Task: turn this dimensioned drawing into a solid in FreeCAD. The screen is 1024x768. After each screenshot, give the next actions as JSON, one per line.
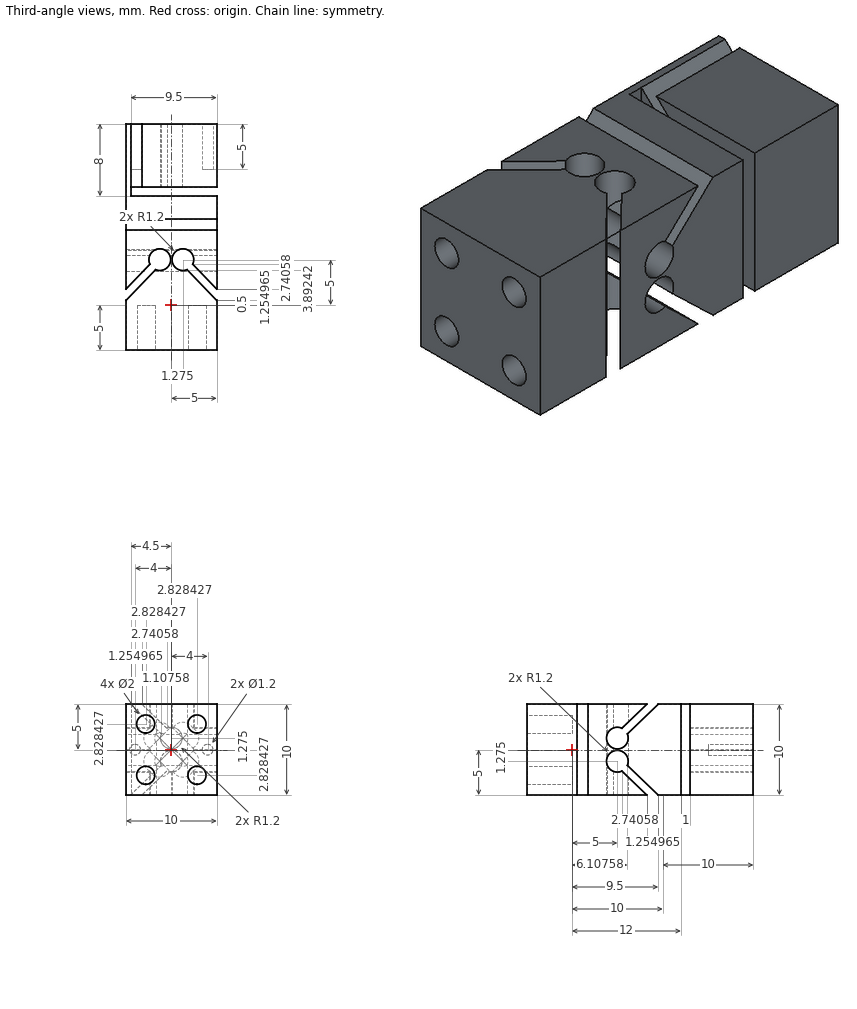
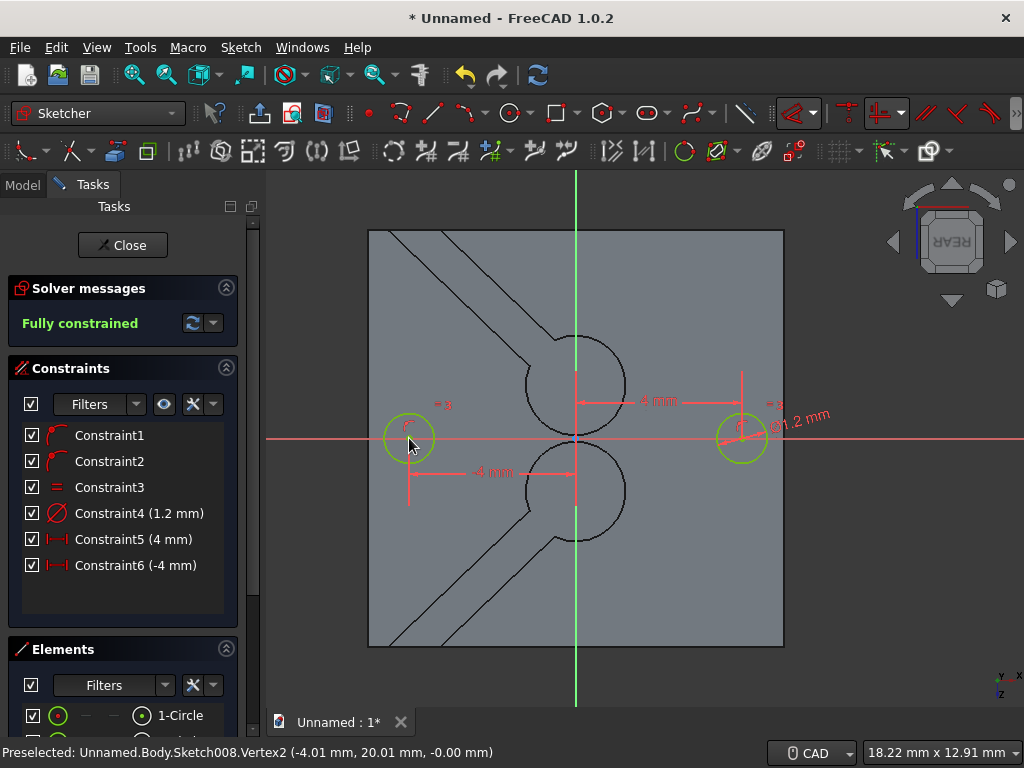
{"action": "left_click", "coordinate": [123, 245]}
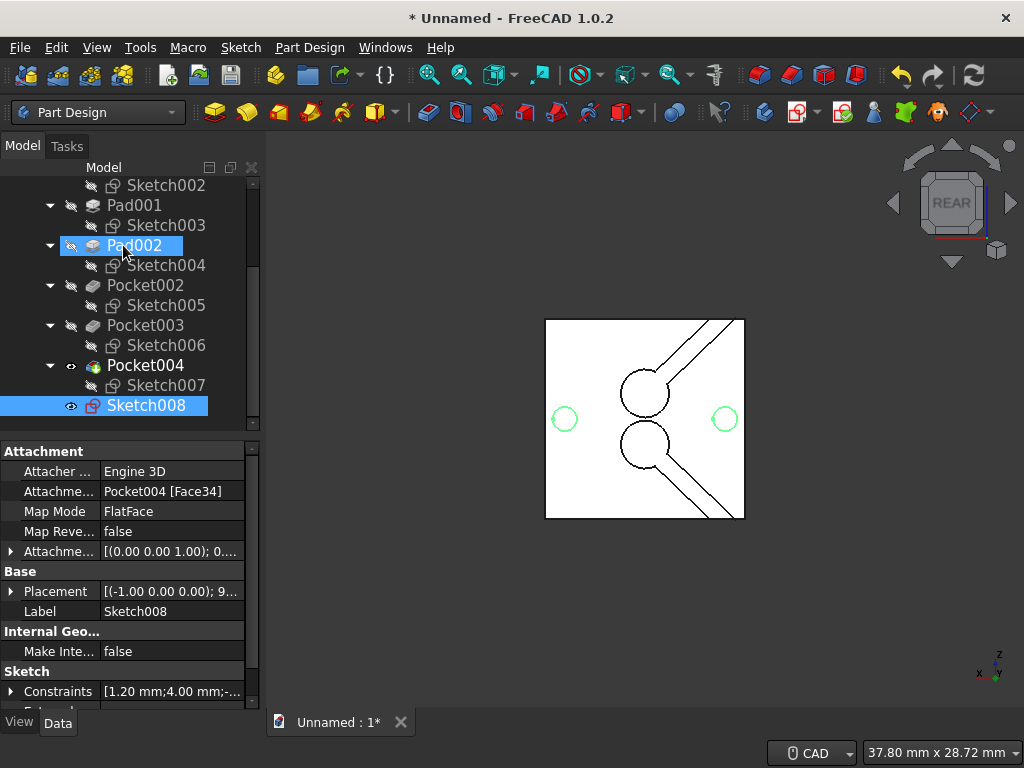
{"action": "left_click", "coordinate": [430, 112]}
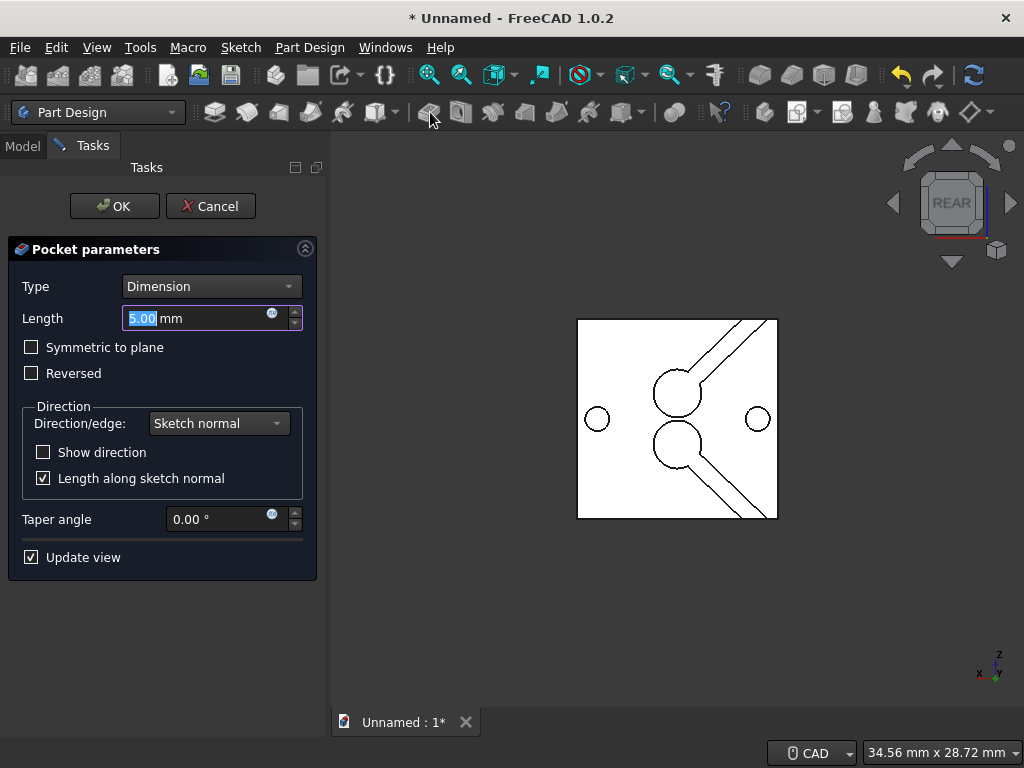
{"action": "type", "text": "5"}
{"action": "key", "text": "Tab"}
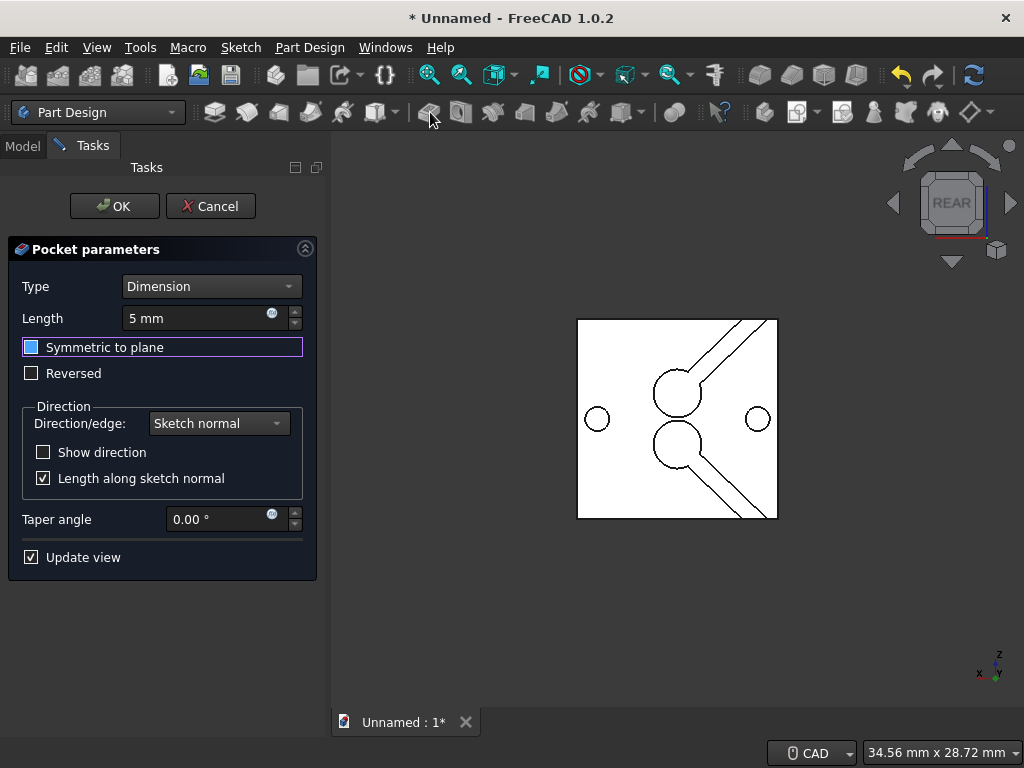
{"action": "left_click", "coordinate": [115, 206]}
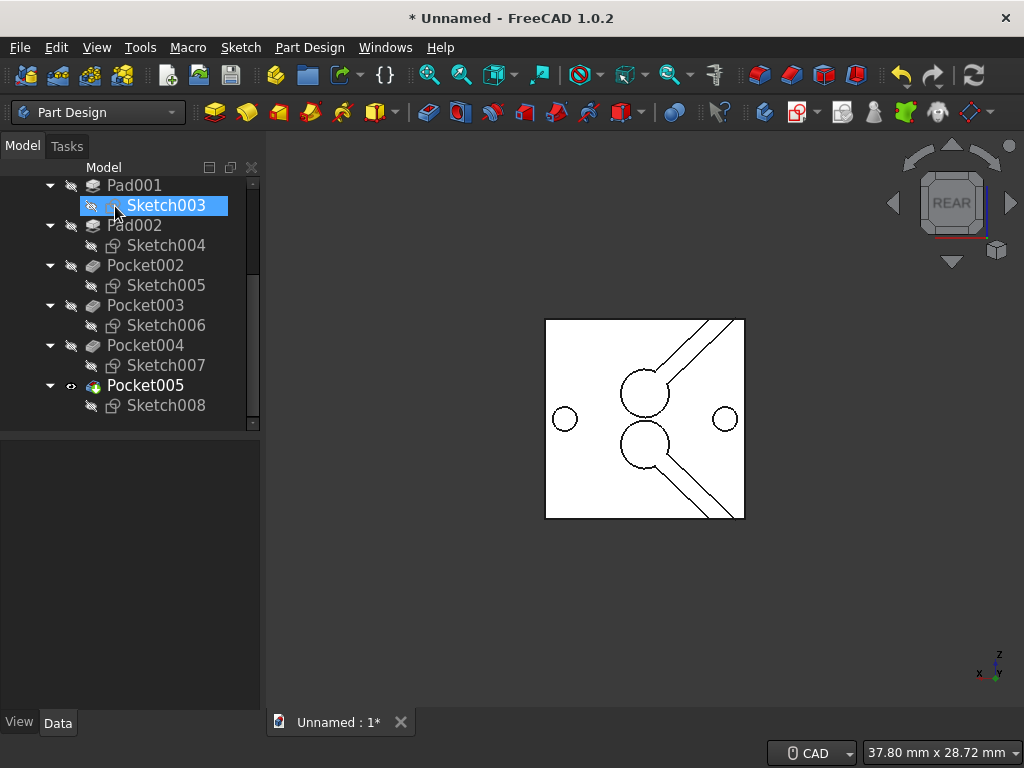
{"action": "key", "text": "0"}